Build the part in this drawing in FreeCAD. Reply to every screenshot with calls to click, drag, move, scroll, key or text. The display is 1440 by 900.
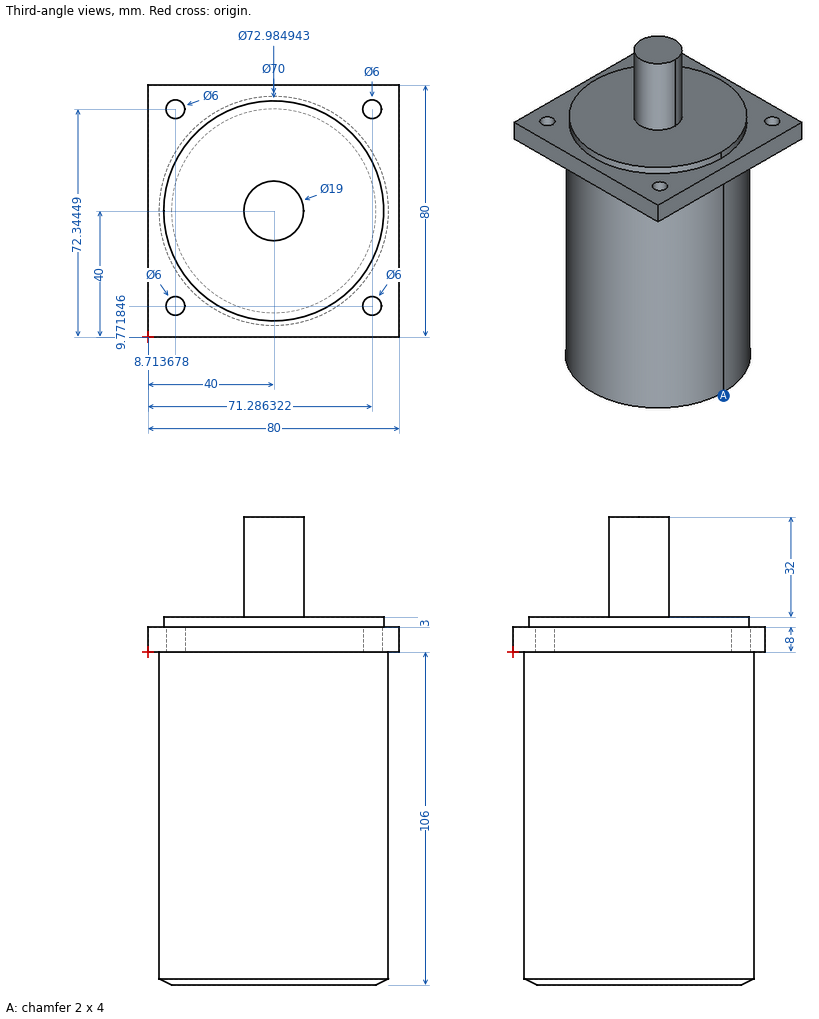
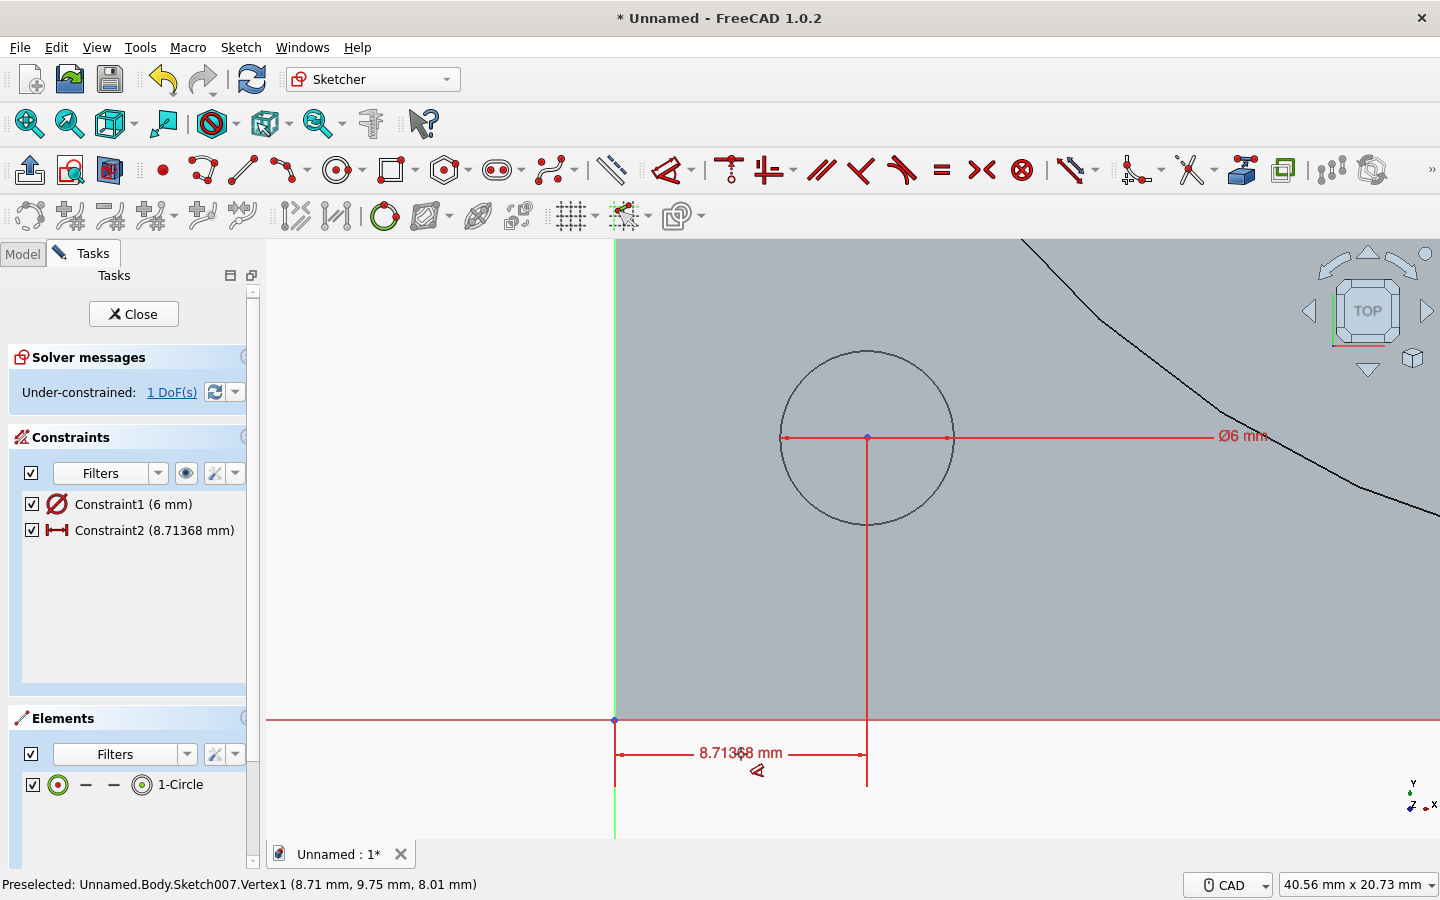
click(867, 438)
click(581, 579)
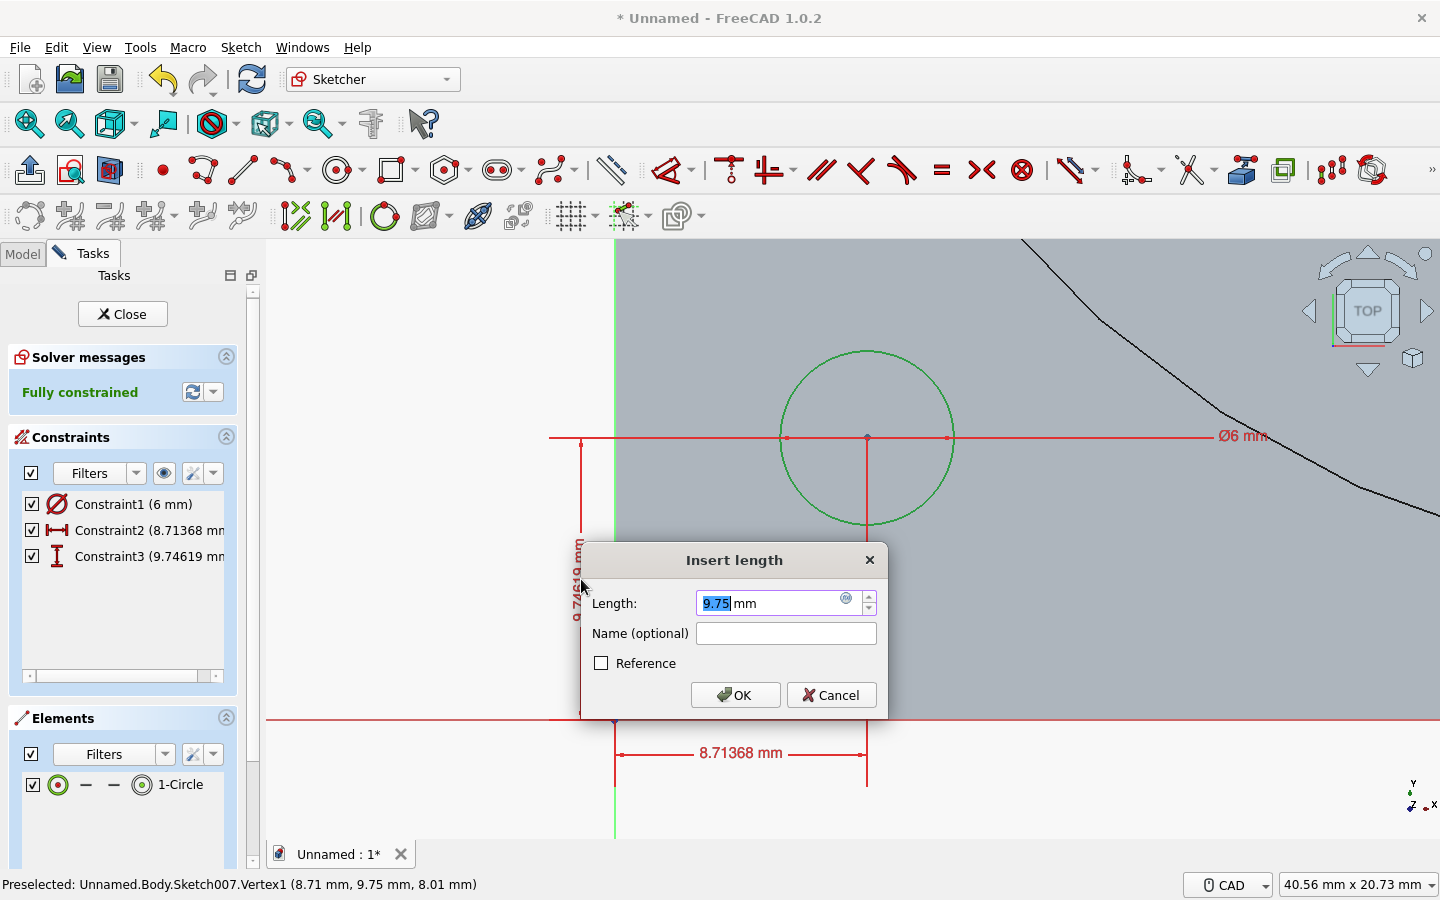
text(9.771846)
key(Return)
key(Escape)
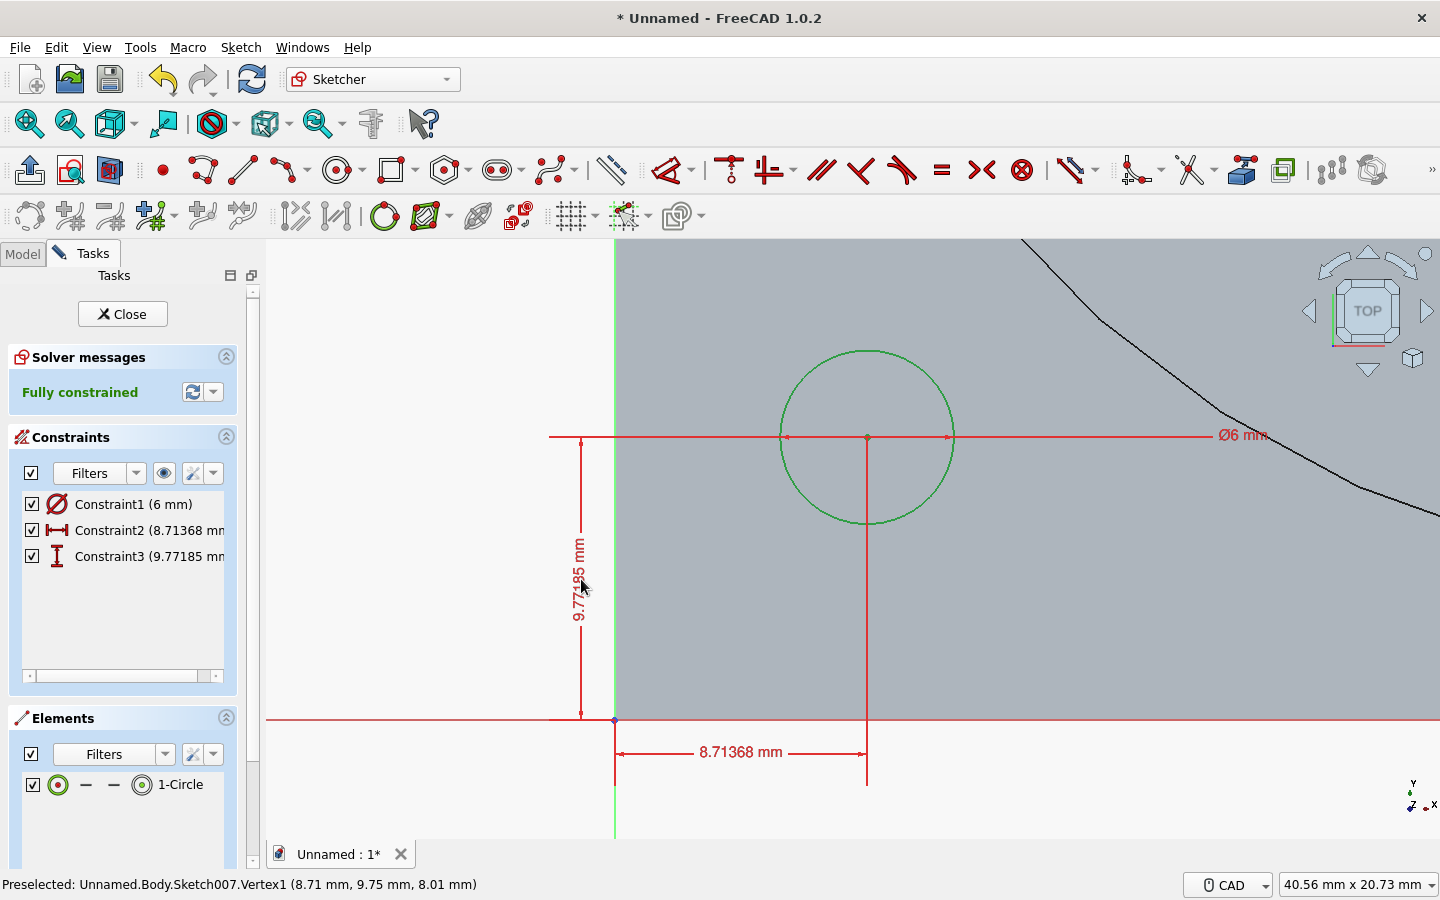
click(123, 314)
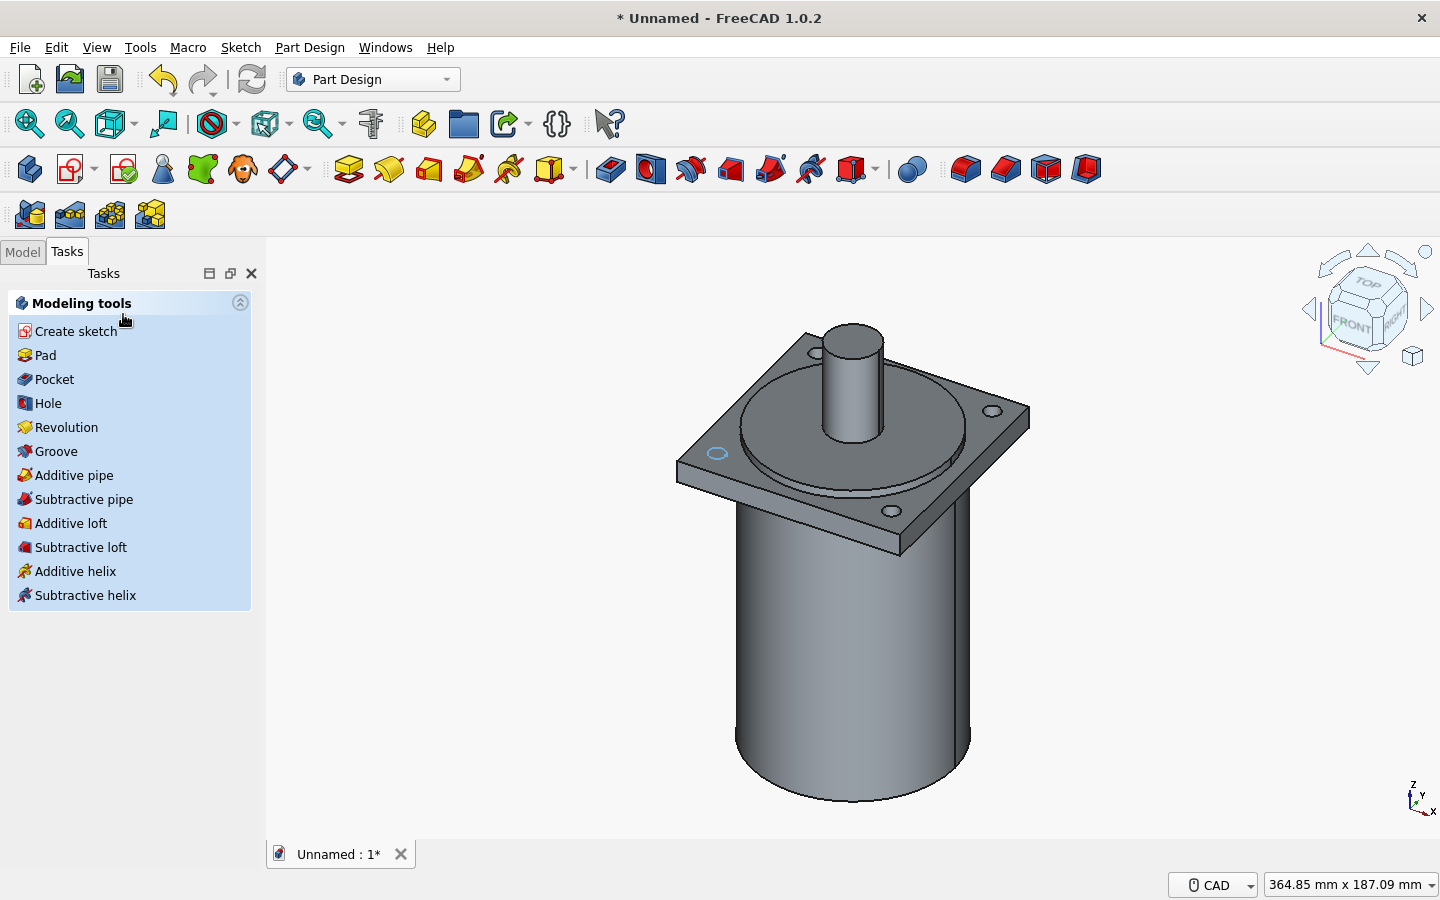
click(612, 170)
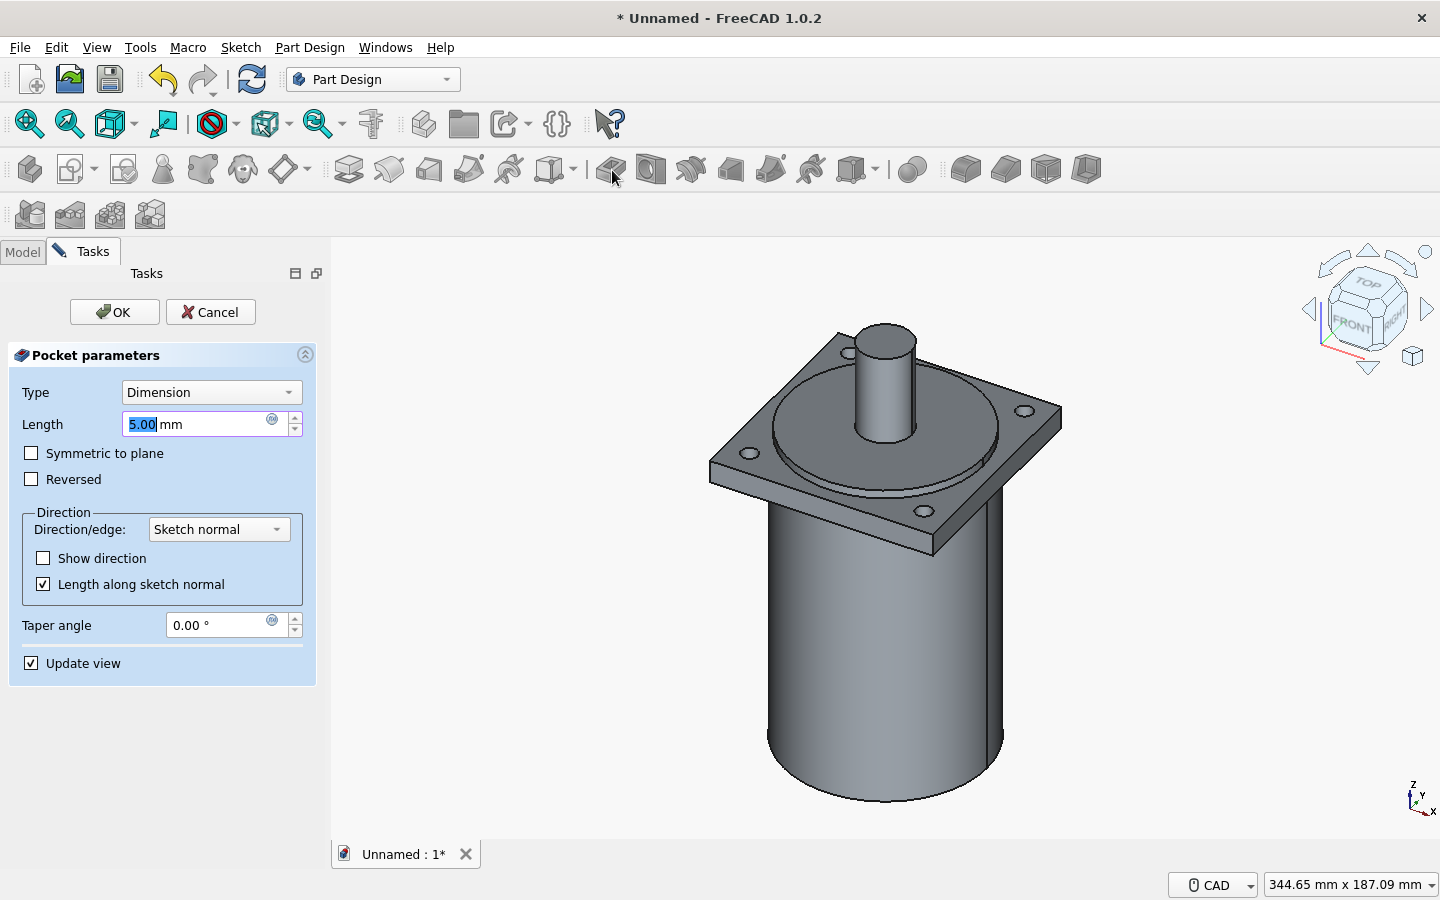
click(212, 392)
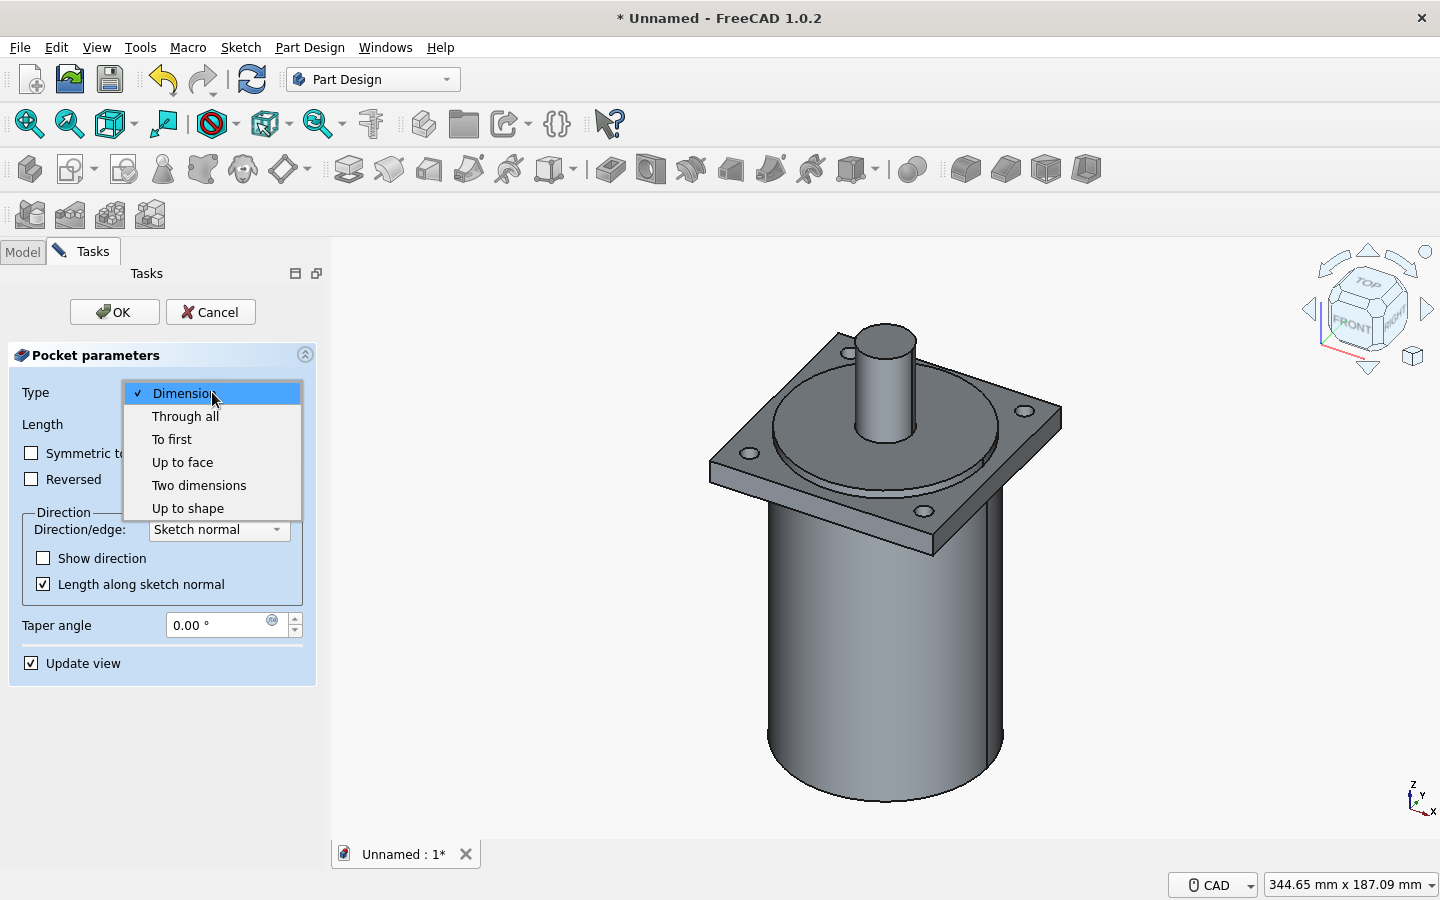
click(212, 440)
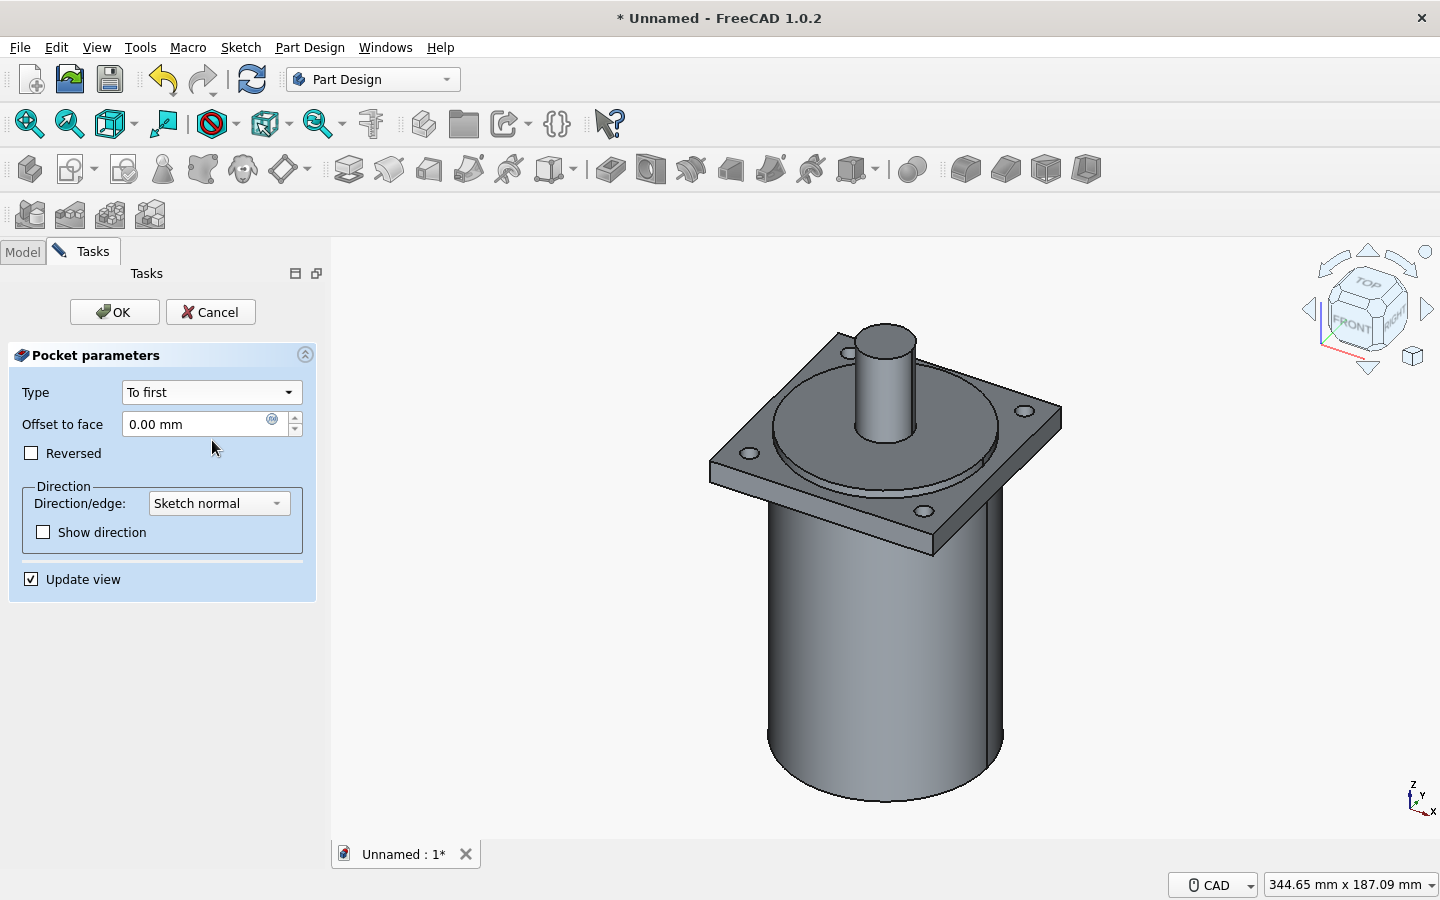
click(115, 312)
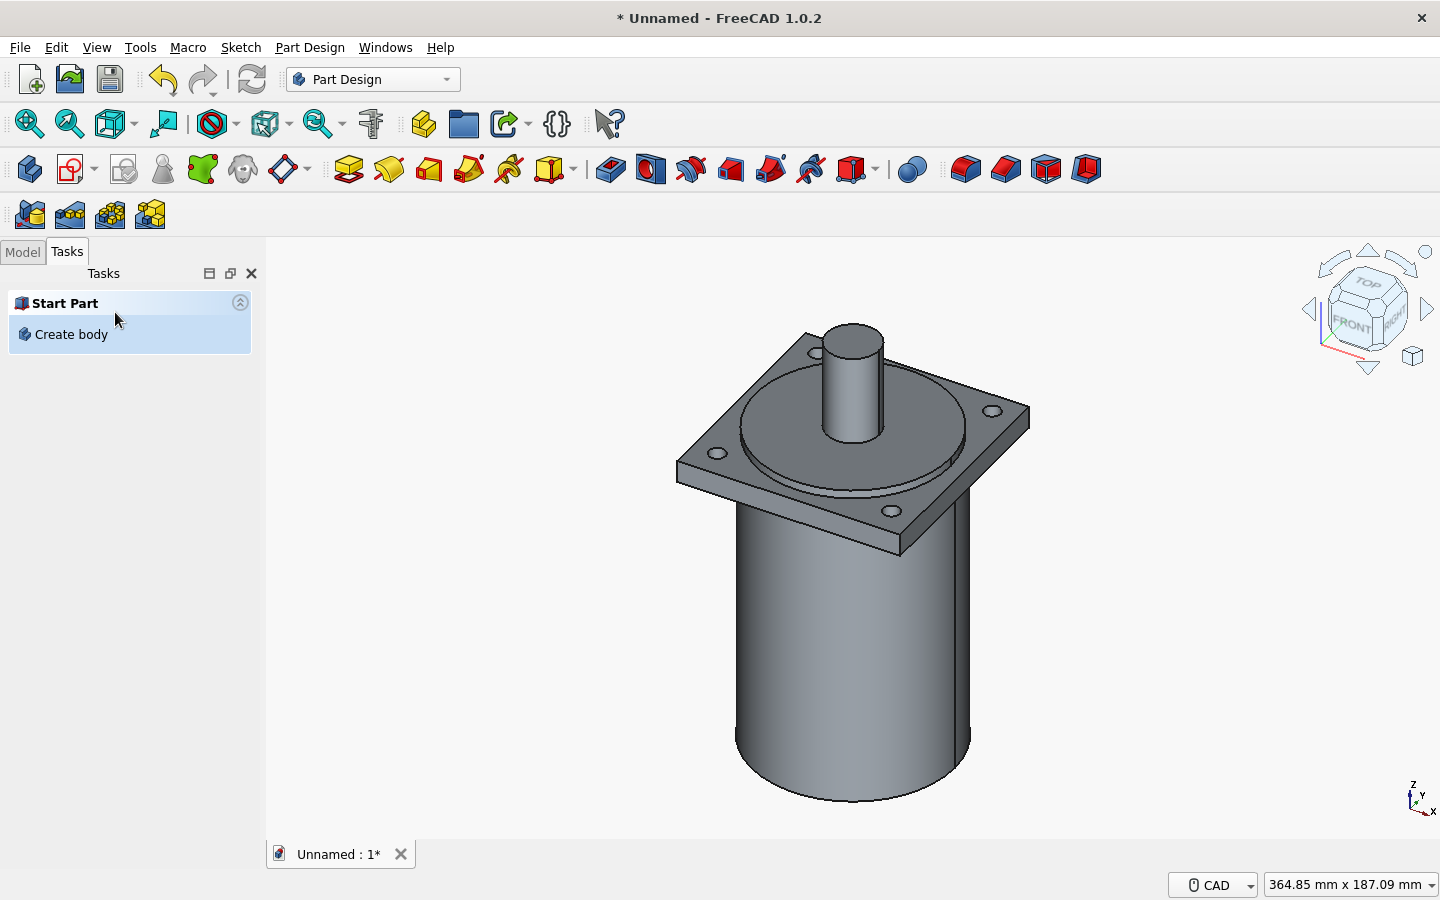
click(964, 756)